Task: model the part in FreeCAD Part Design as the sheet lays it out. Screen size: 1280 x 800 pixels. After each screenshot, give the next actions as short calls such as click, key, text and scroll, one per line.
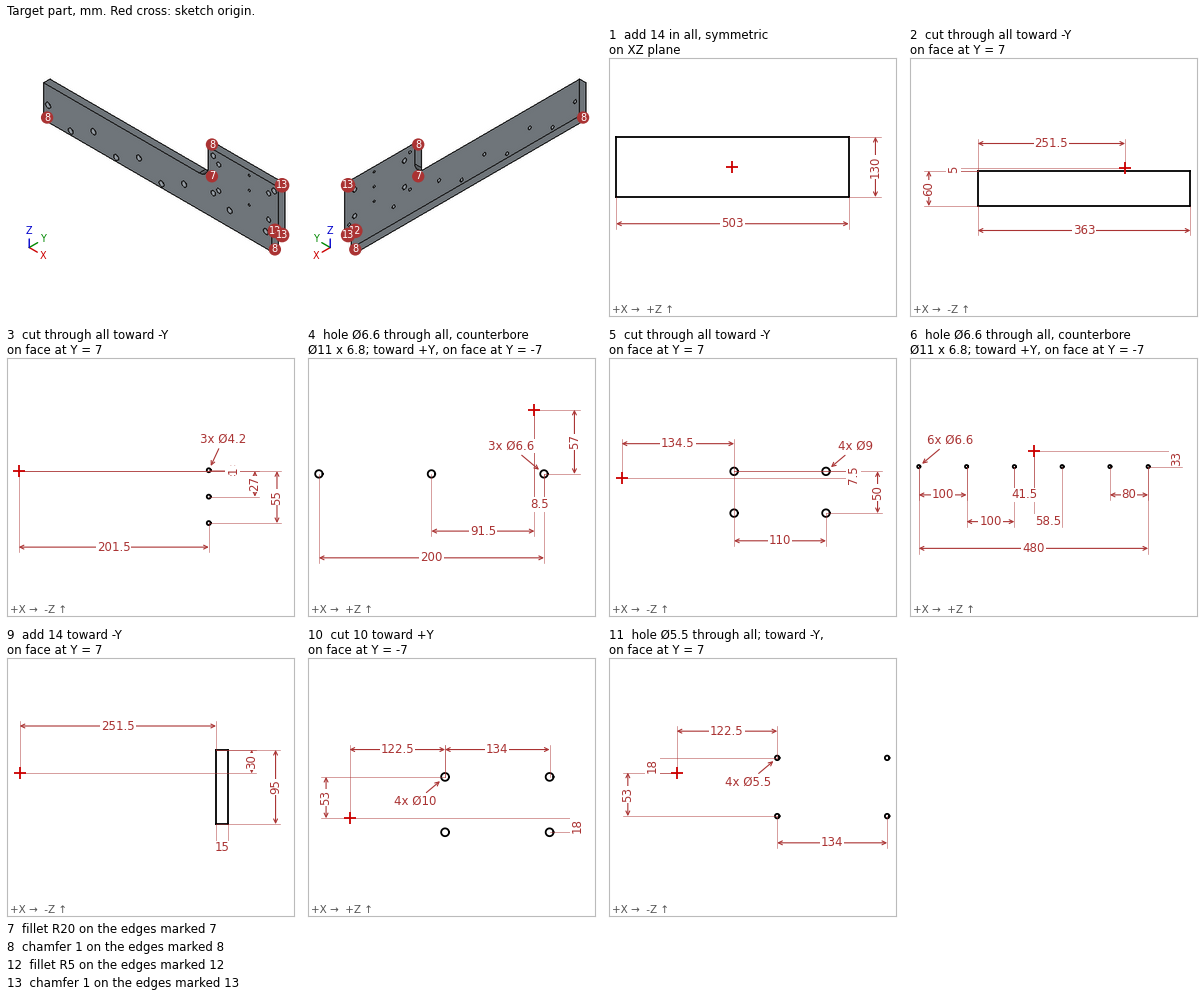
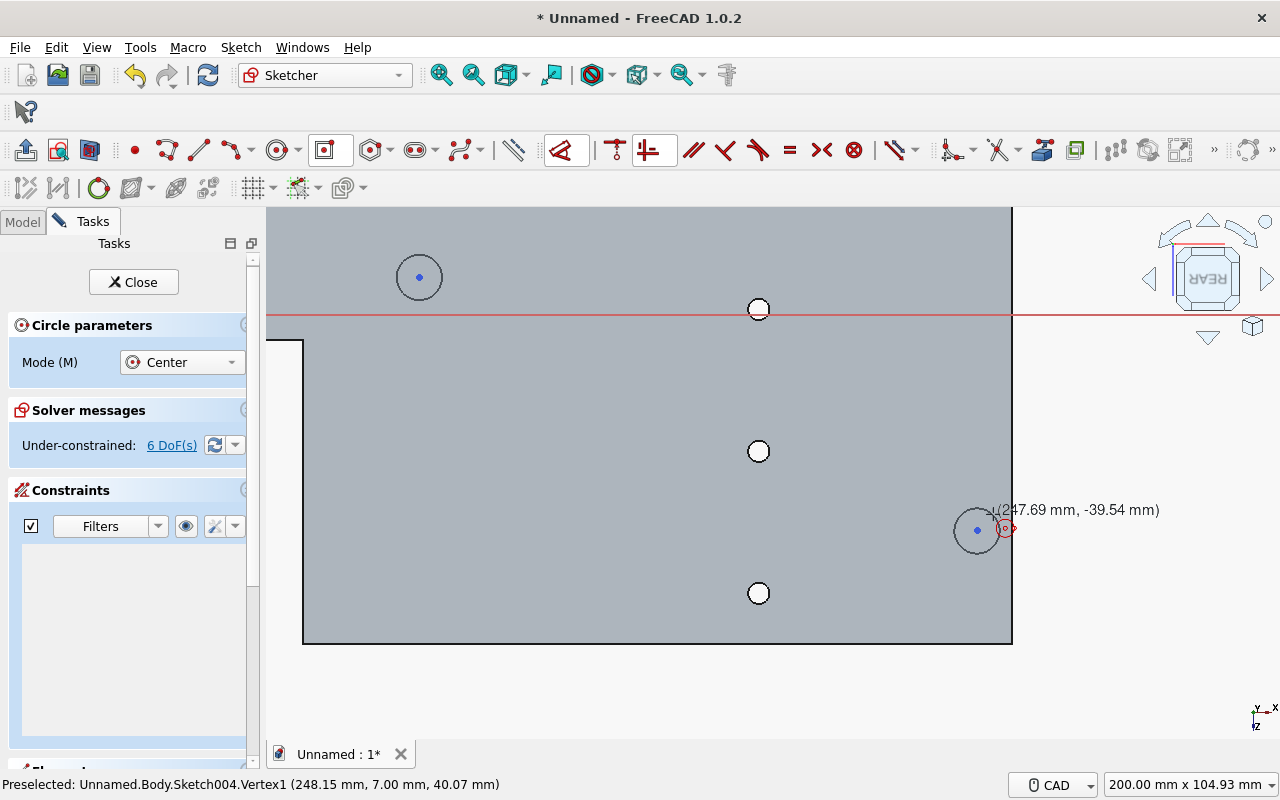
click(419, 530)
click(435, 514)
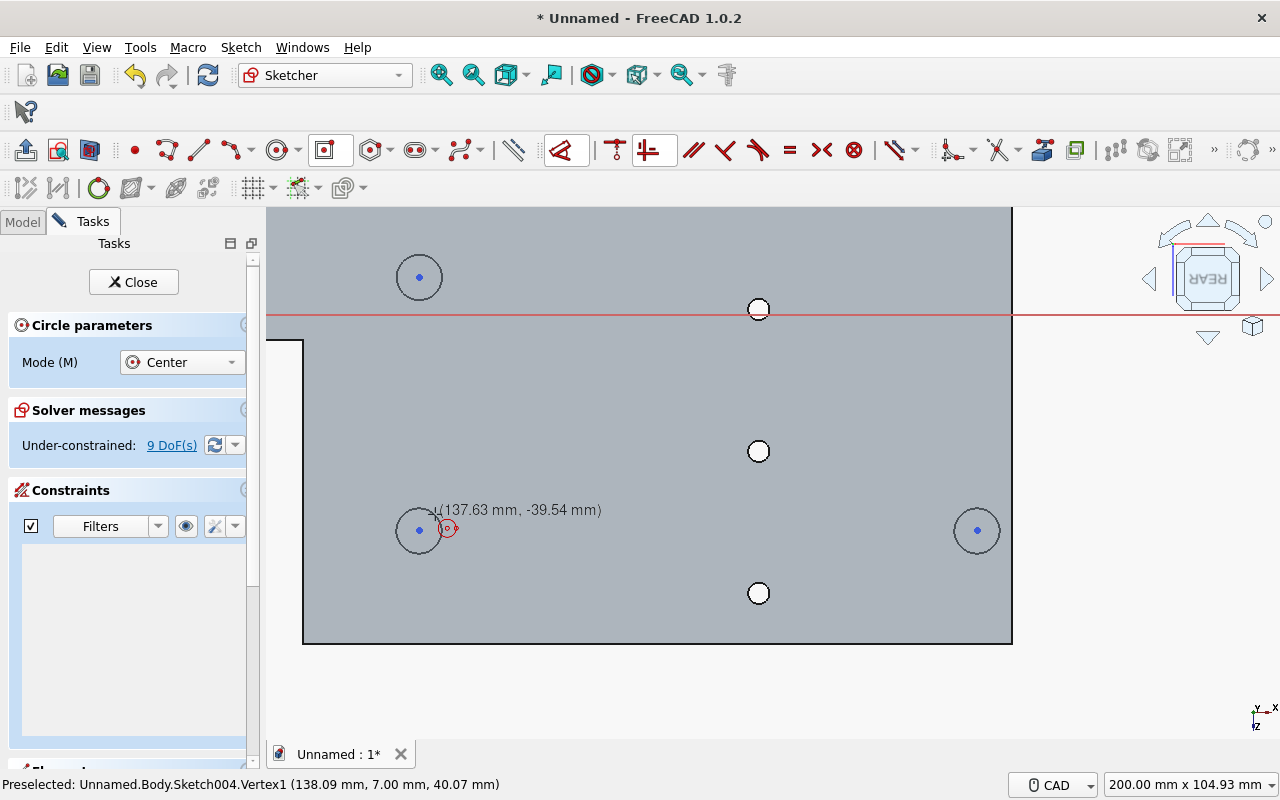
click(977, 277)
click(993, 260)
key(Escape)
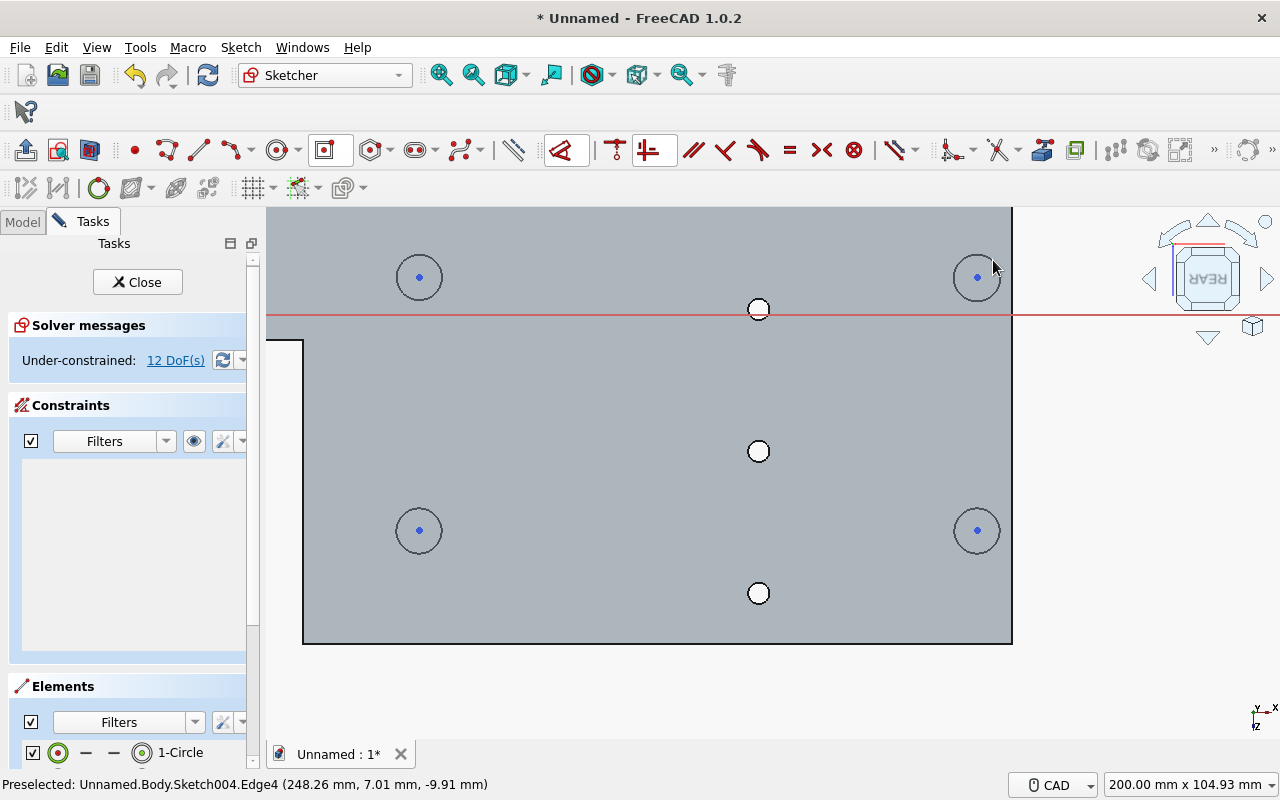
click(435, 261)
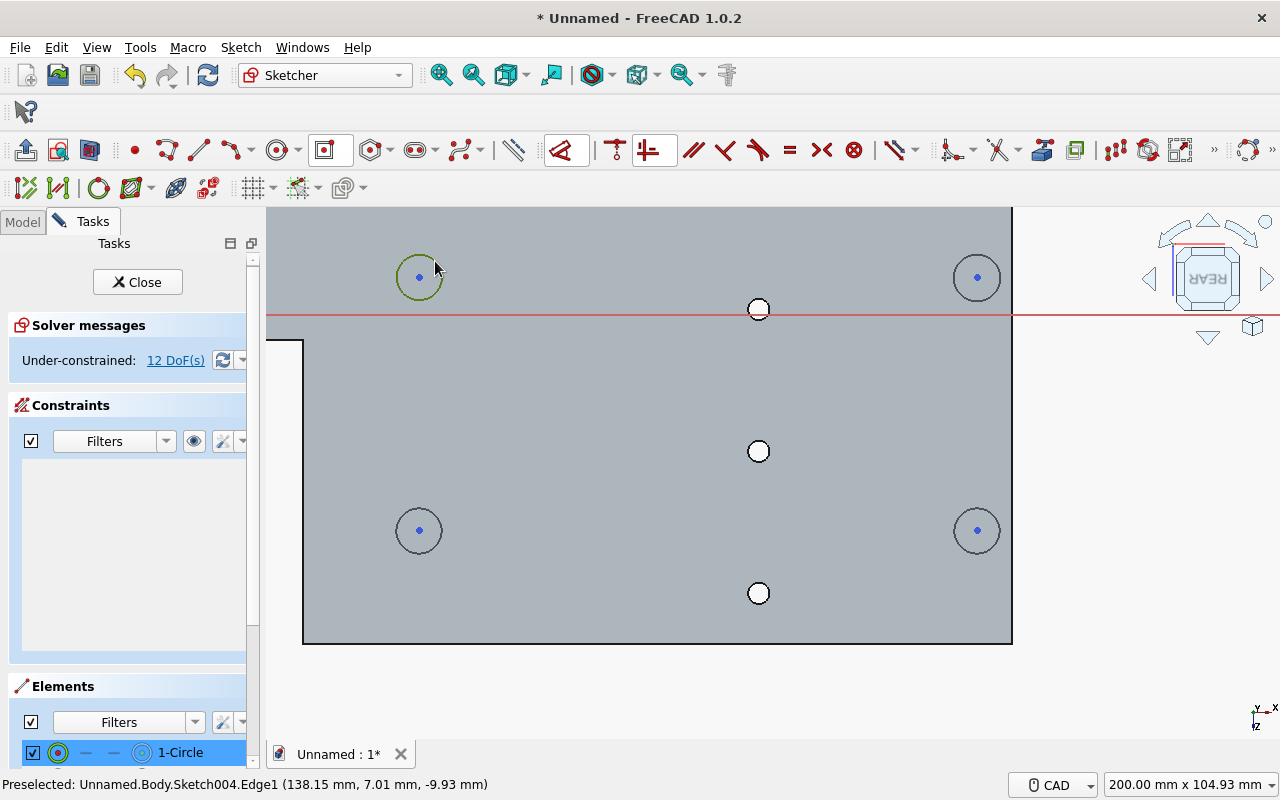
click(993, 515)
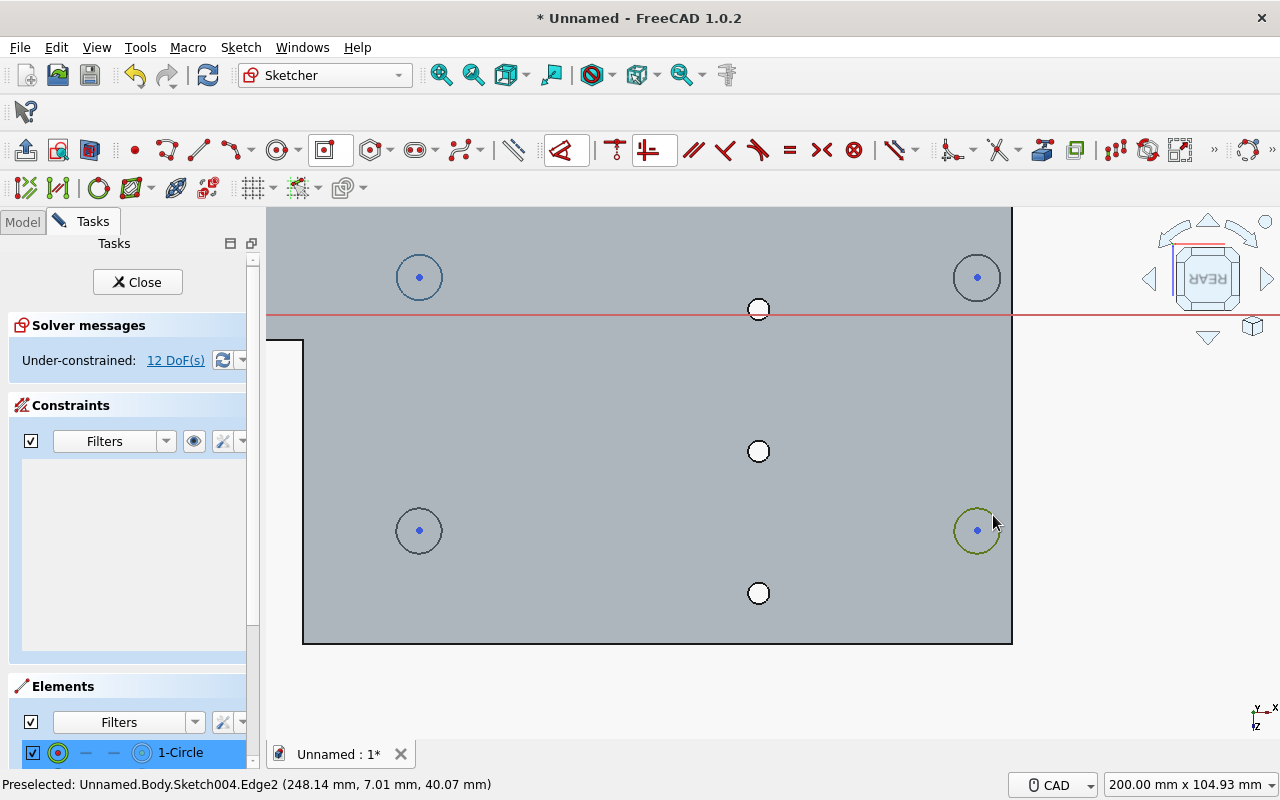
click(435, 515)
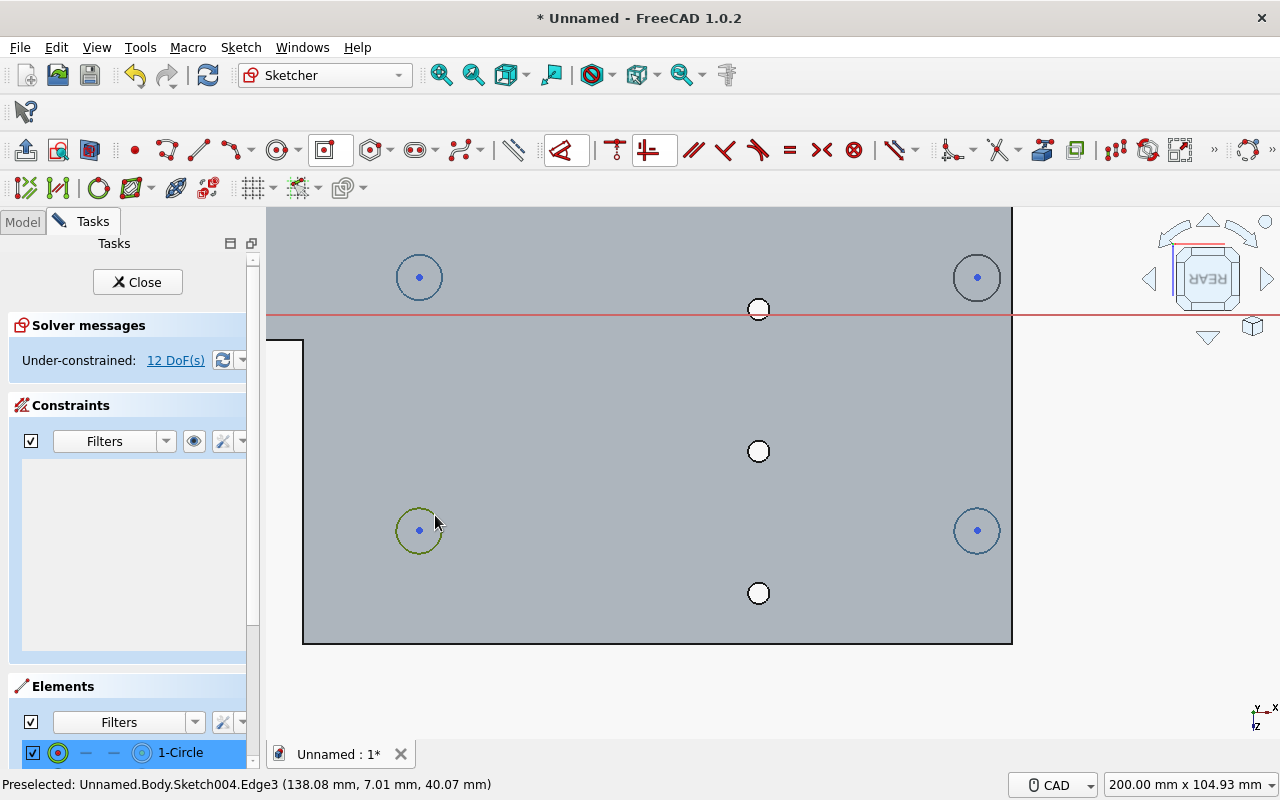
click(993, 261)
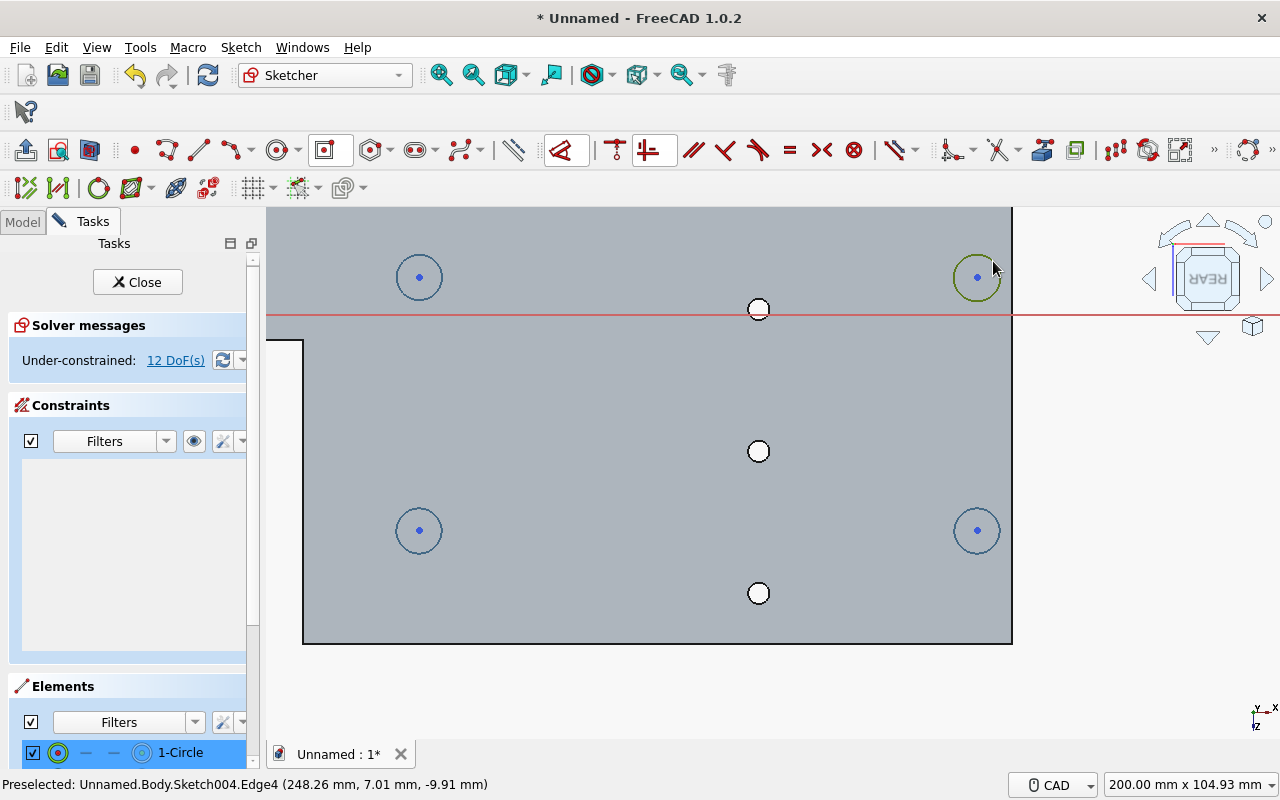
key(e)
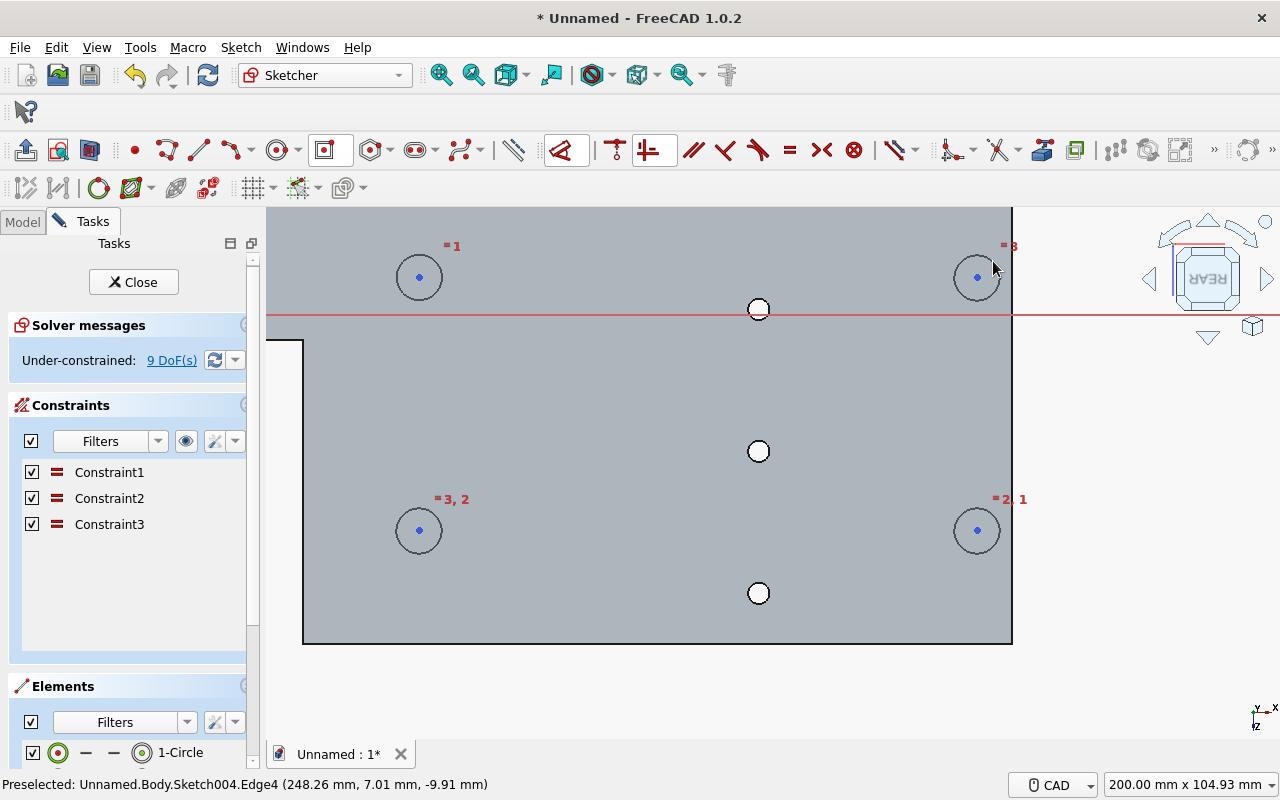
click(419, 277)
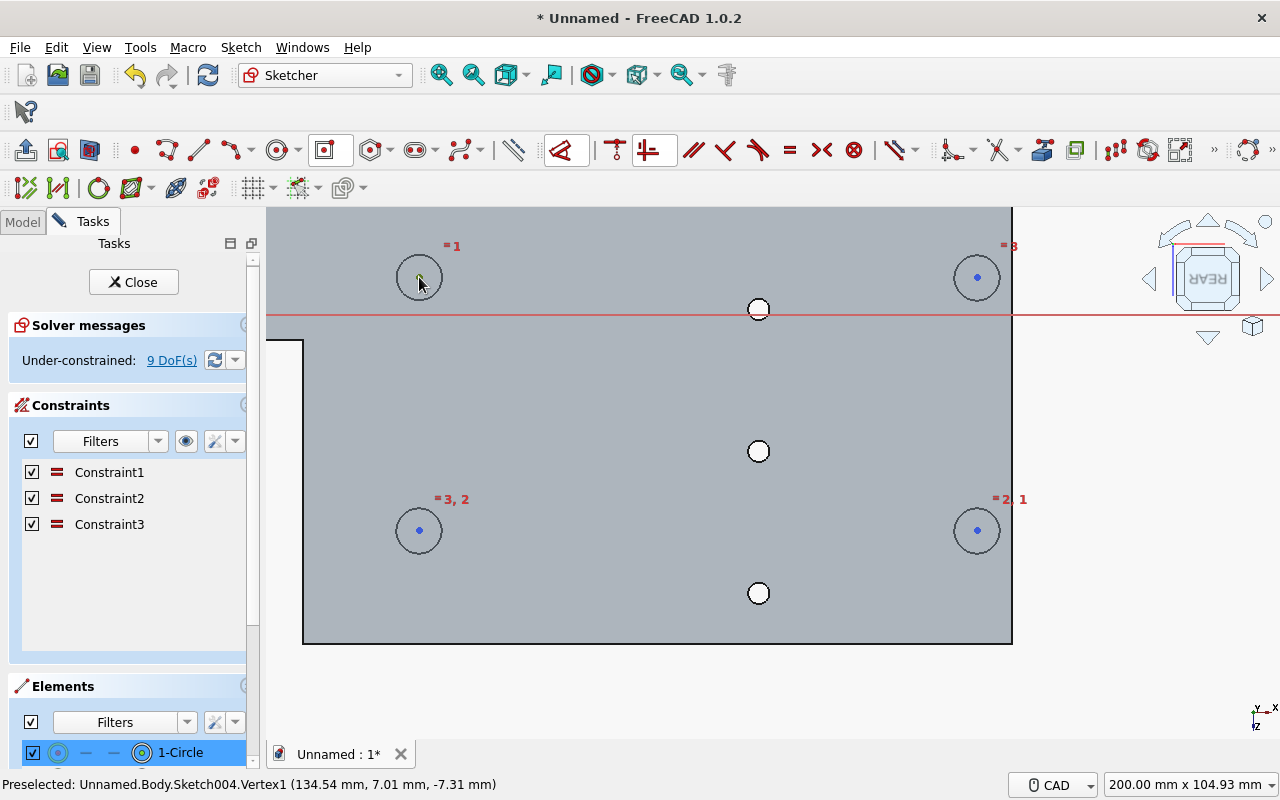
click(419, 531)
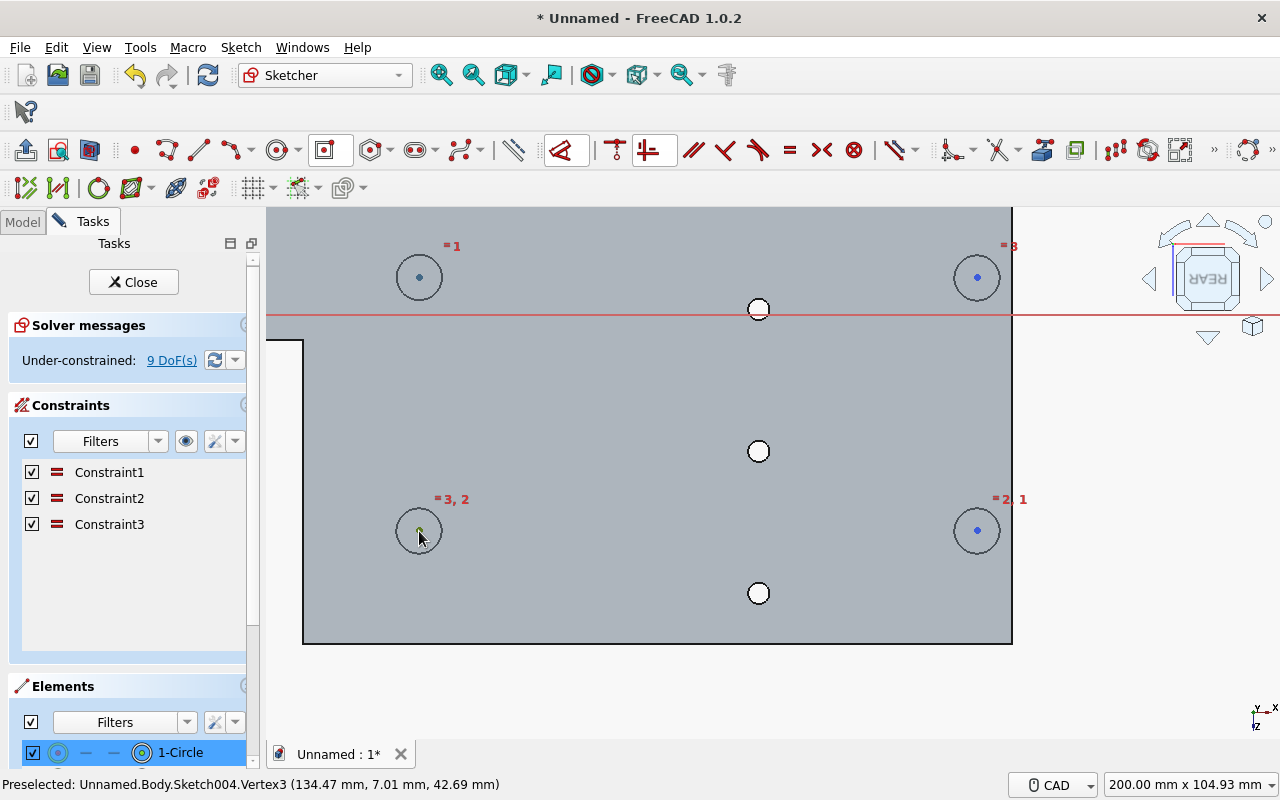
key(v)